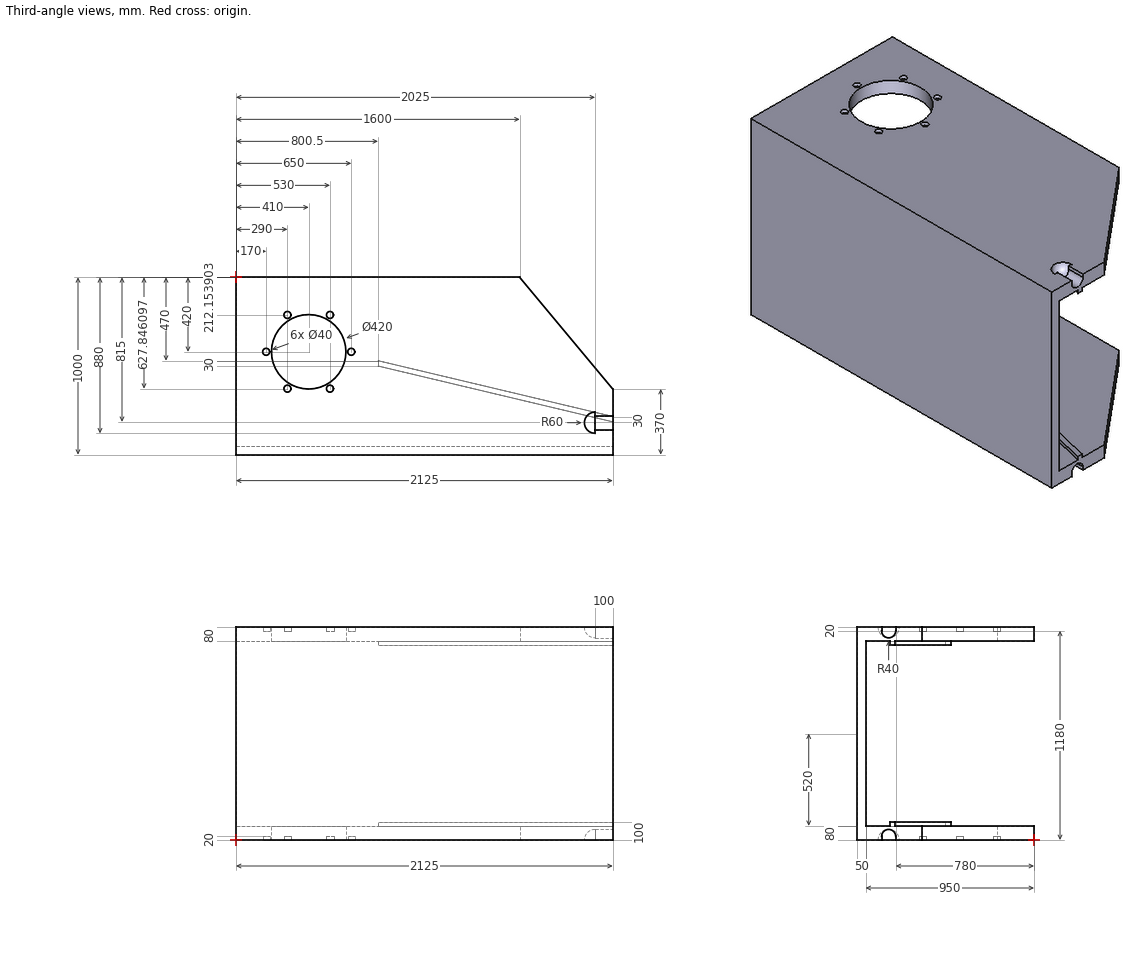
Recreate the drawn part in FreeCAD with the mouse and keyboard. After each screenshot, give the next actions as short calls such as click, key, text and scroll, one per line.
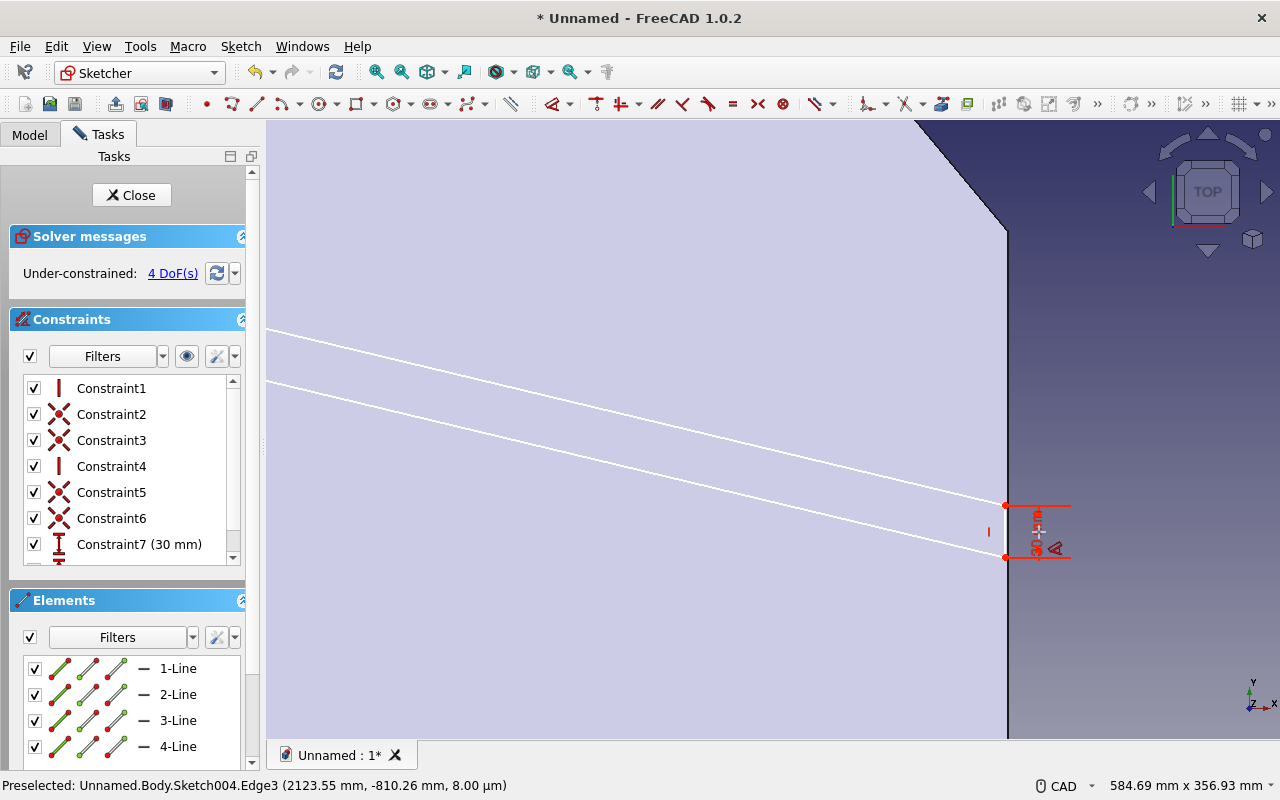
scroll(1009, 545, down, 9)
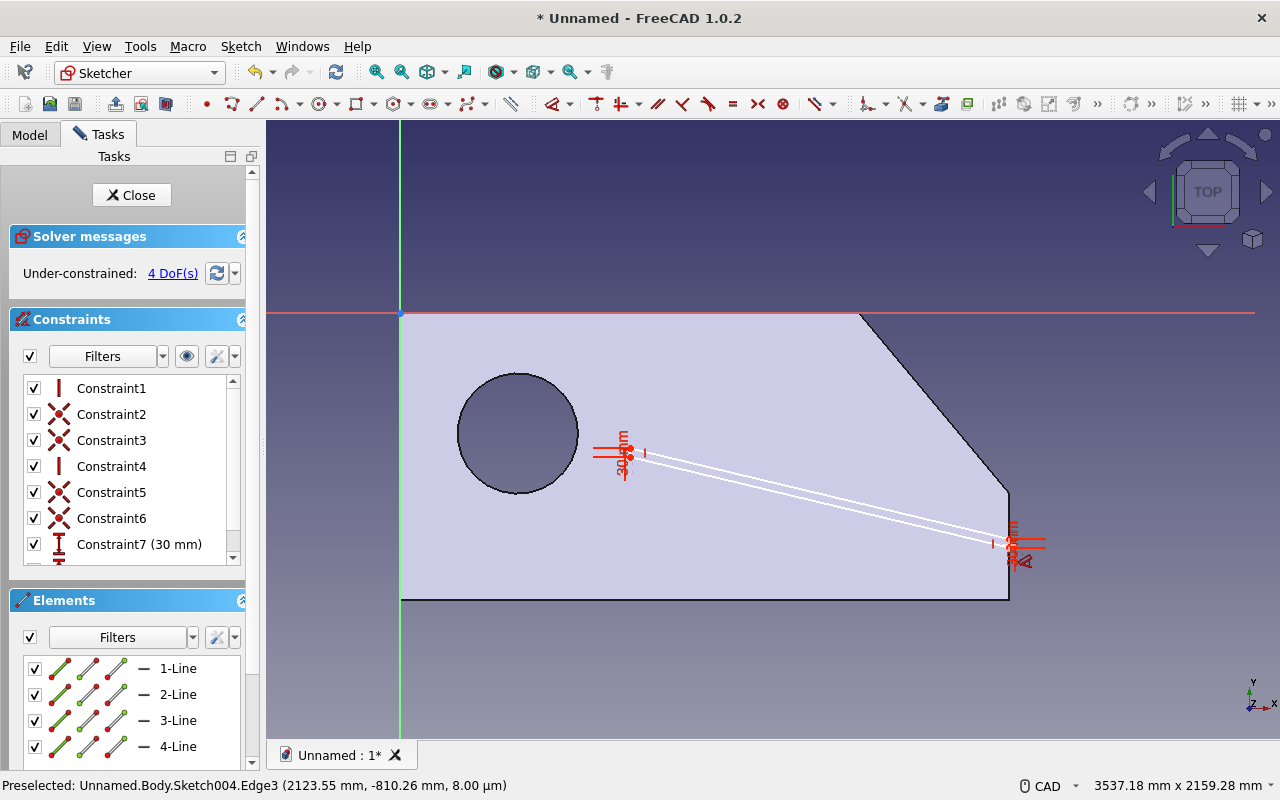
scroll(630, 448, up, 2)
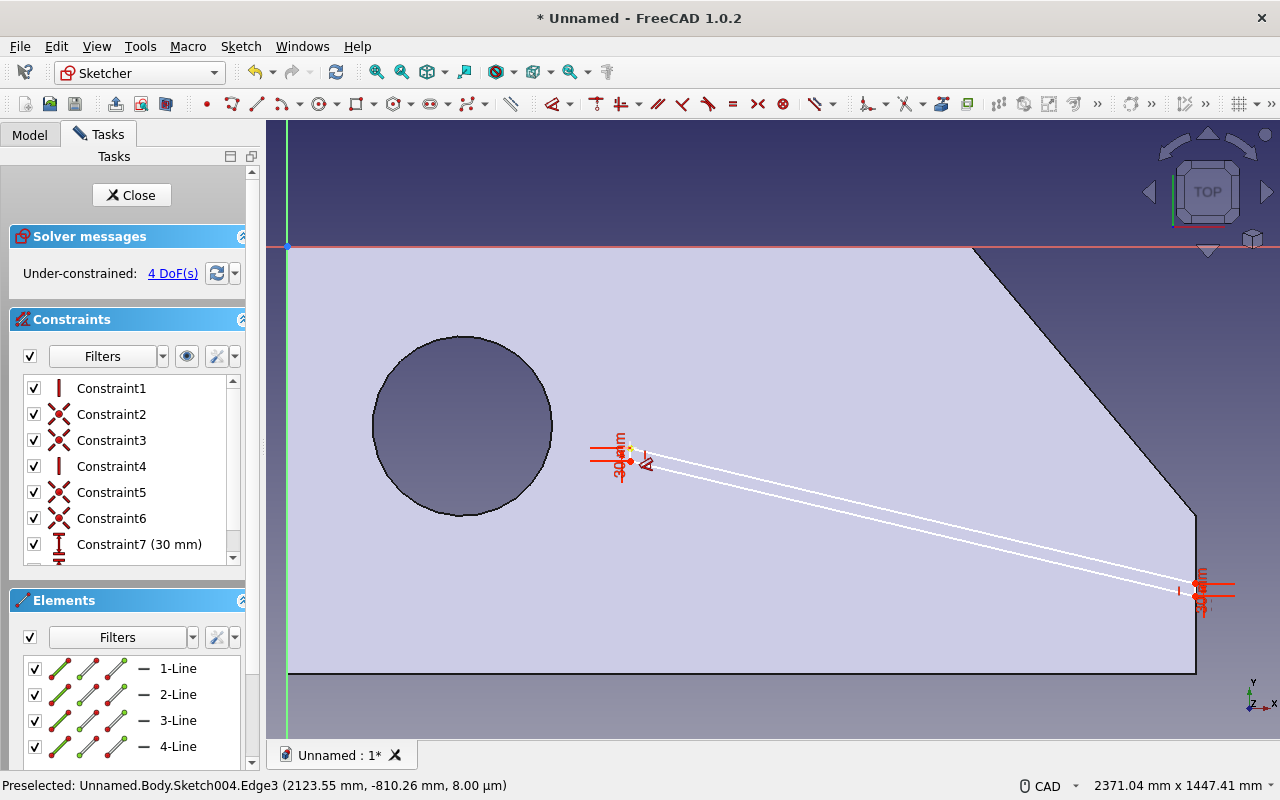
click(630, 448)
click(664, 347)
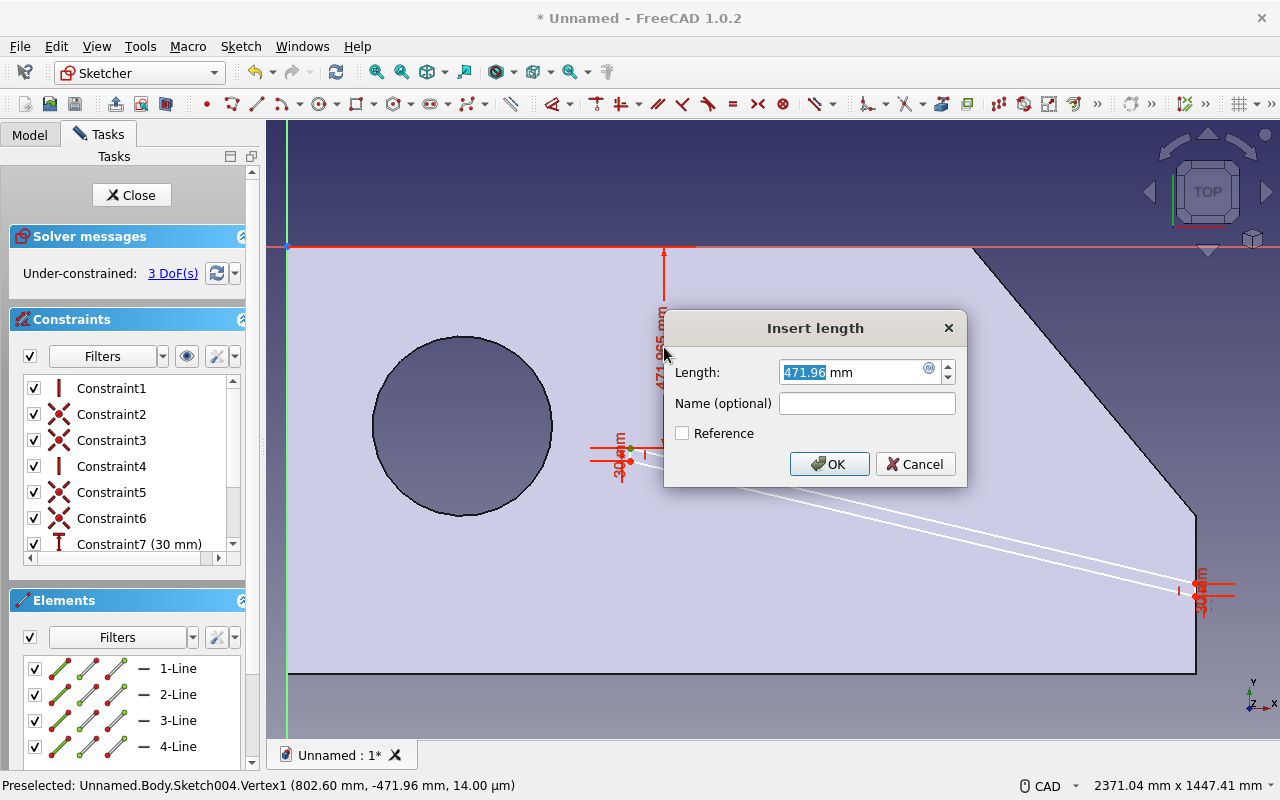
text(470)
key(Return)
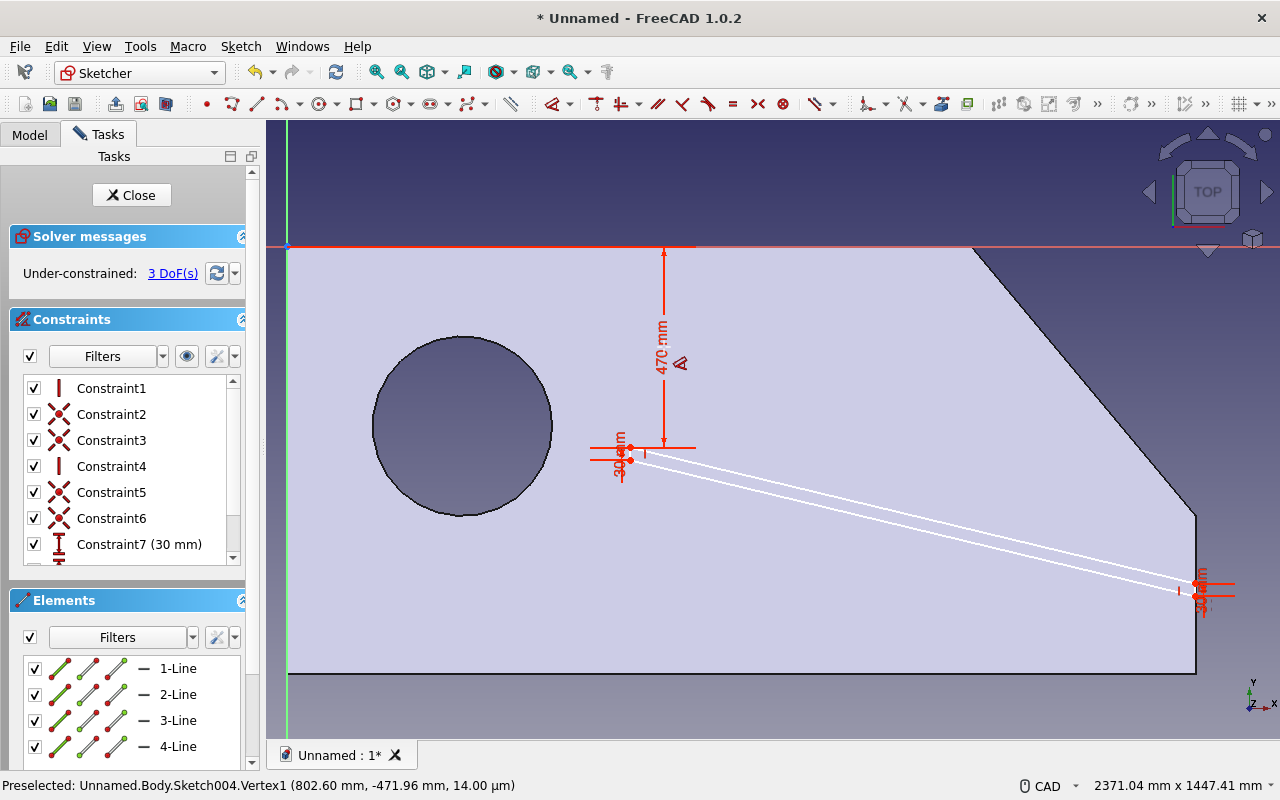
scroll(629, 447, down, 2)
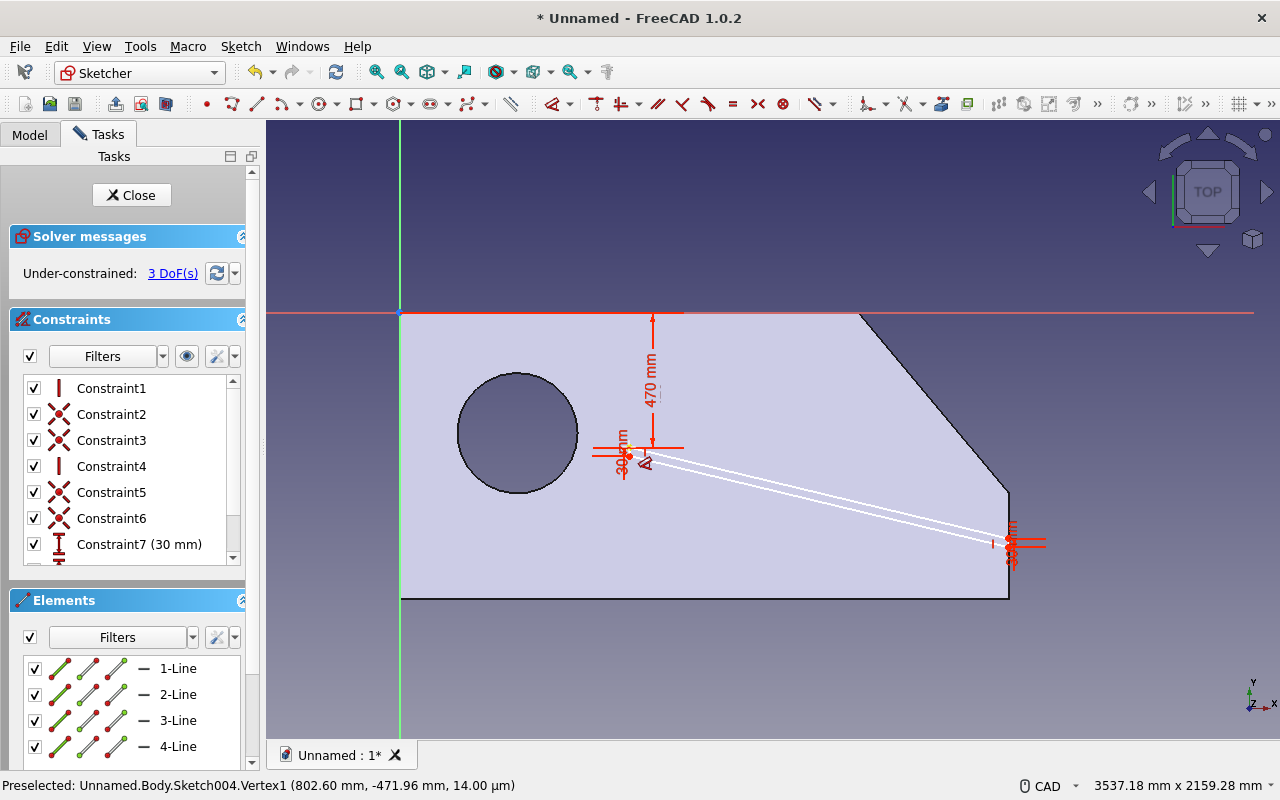
scroll(1009, 547, up, 2)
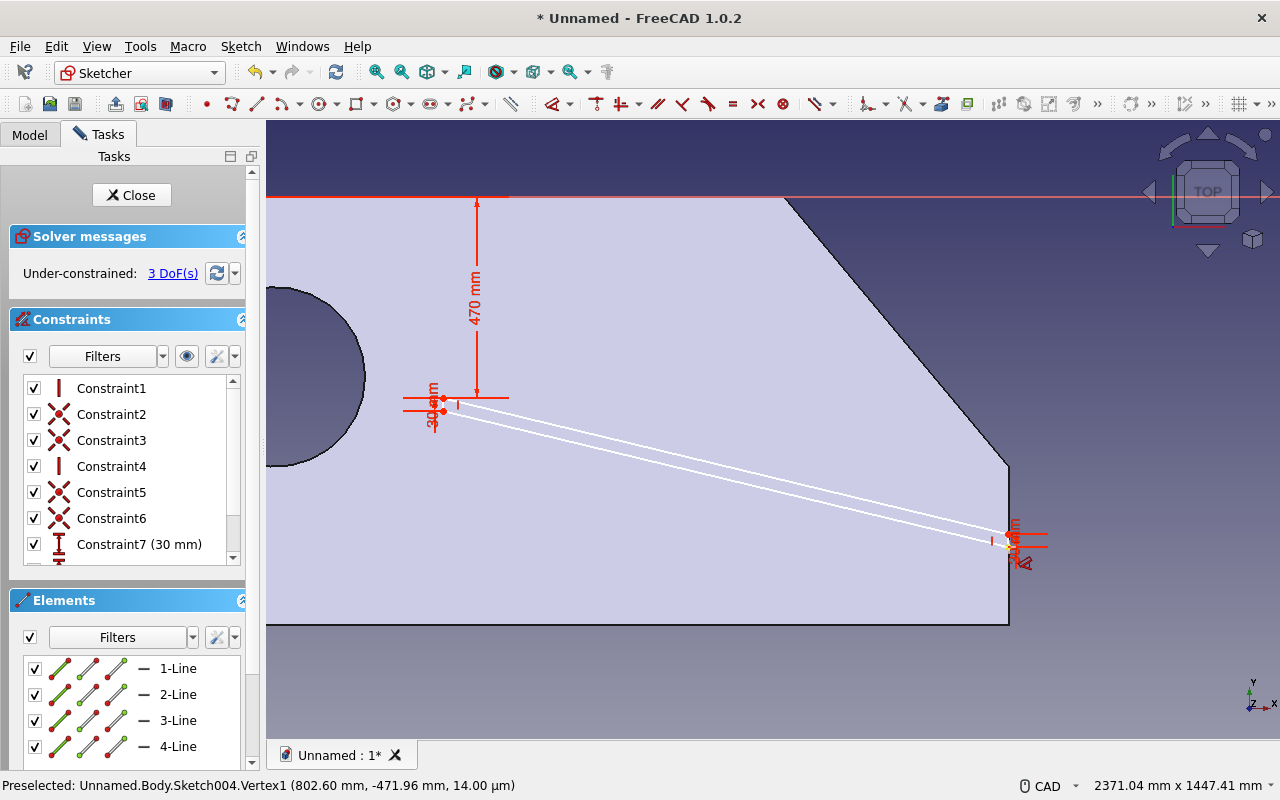
click(1008, 547)
click(1042, 372)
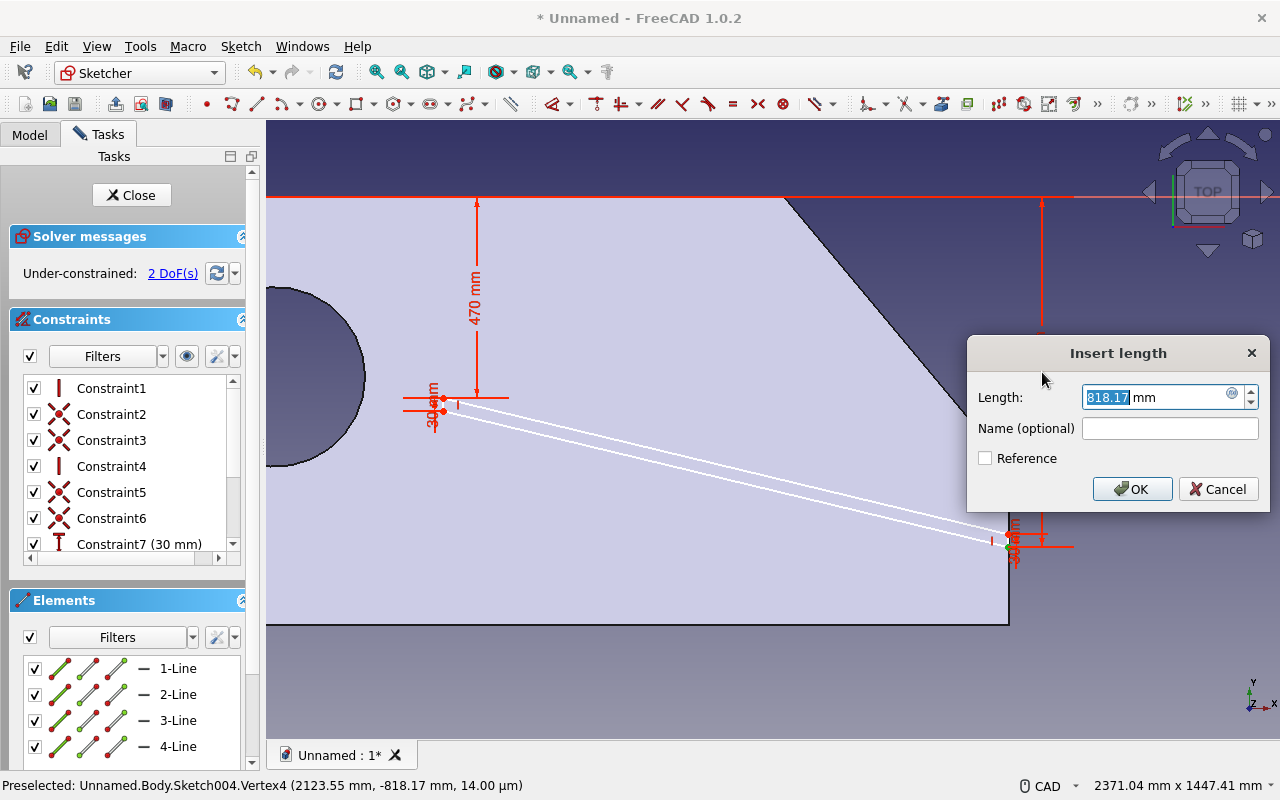
text(815)
key(Return)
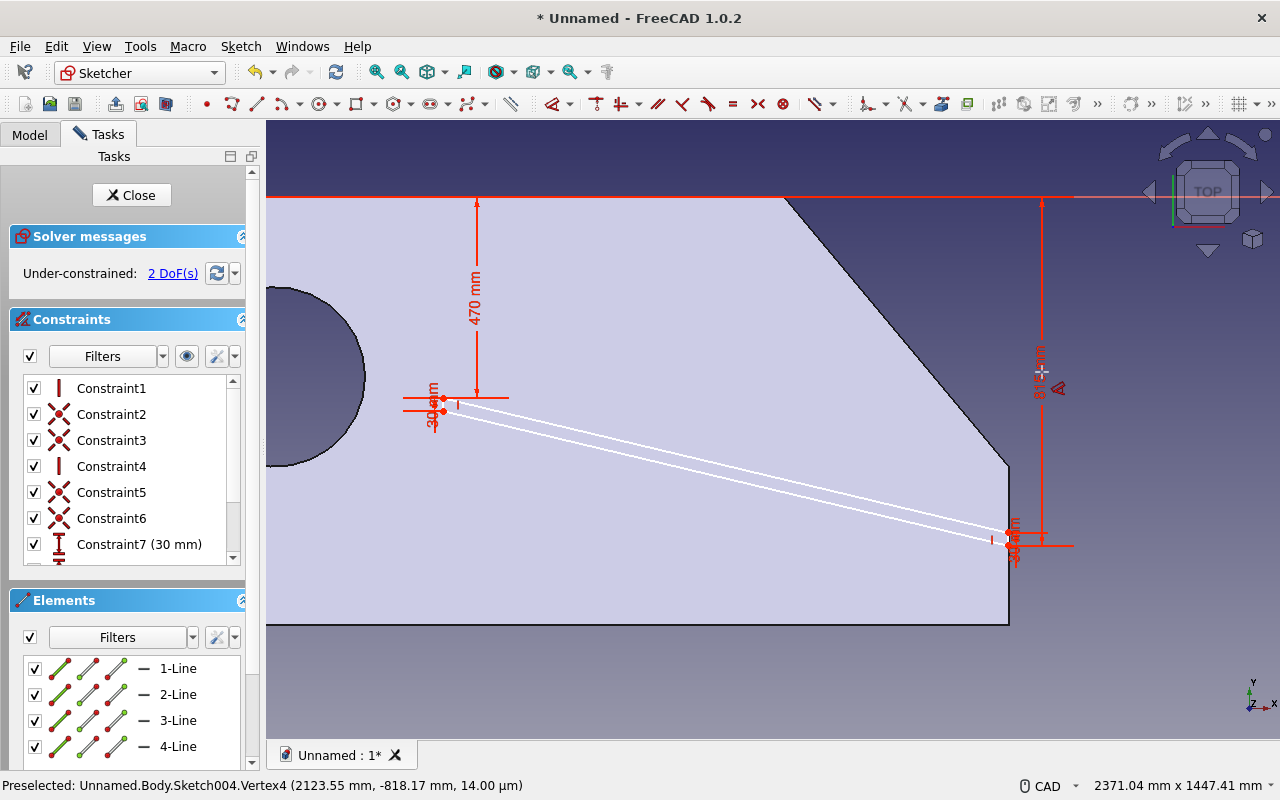
click(1008, 546)
click(651, 580)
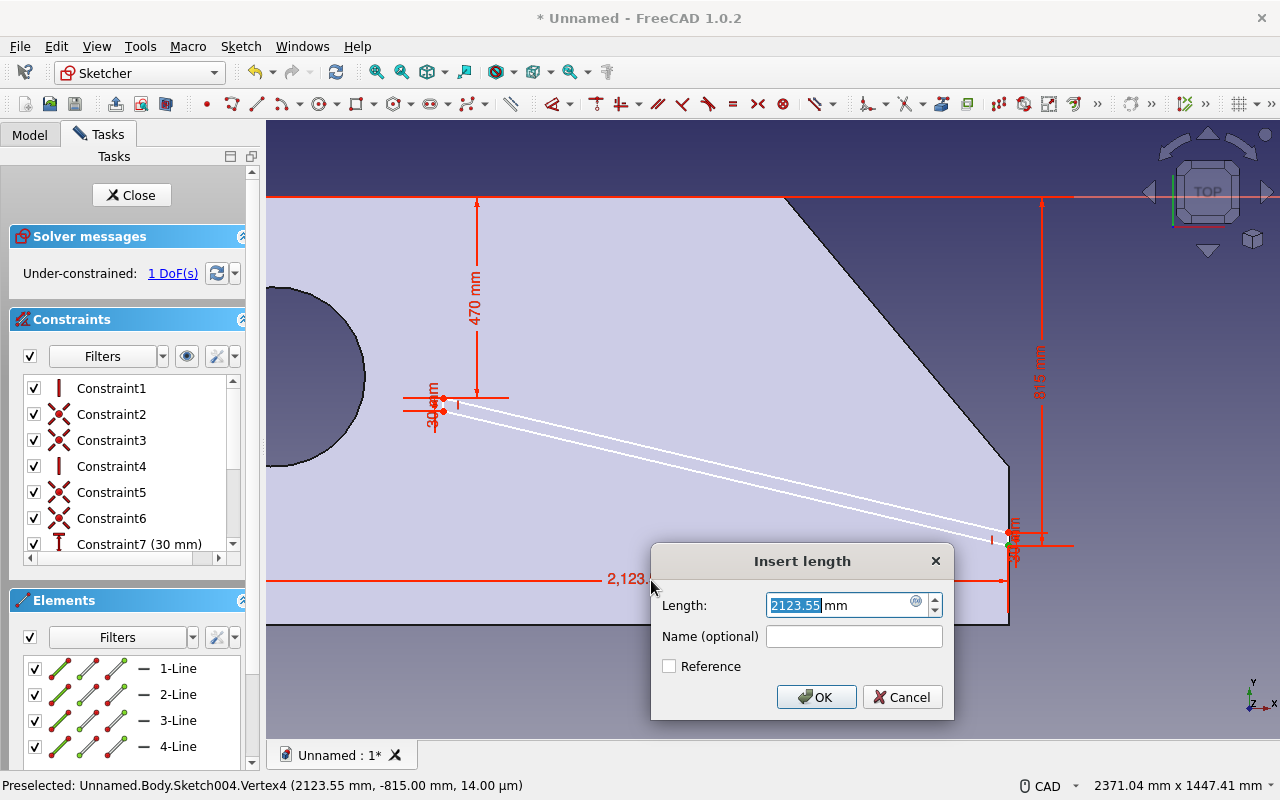
text(2125)
key(Return)